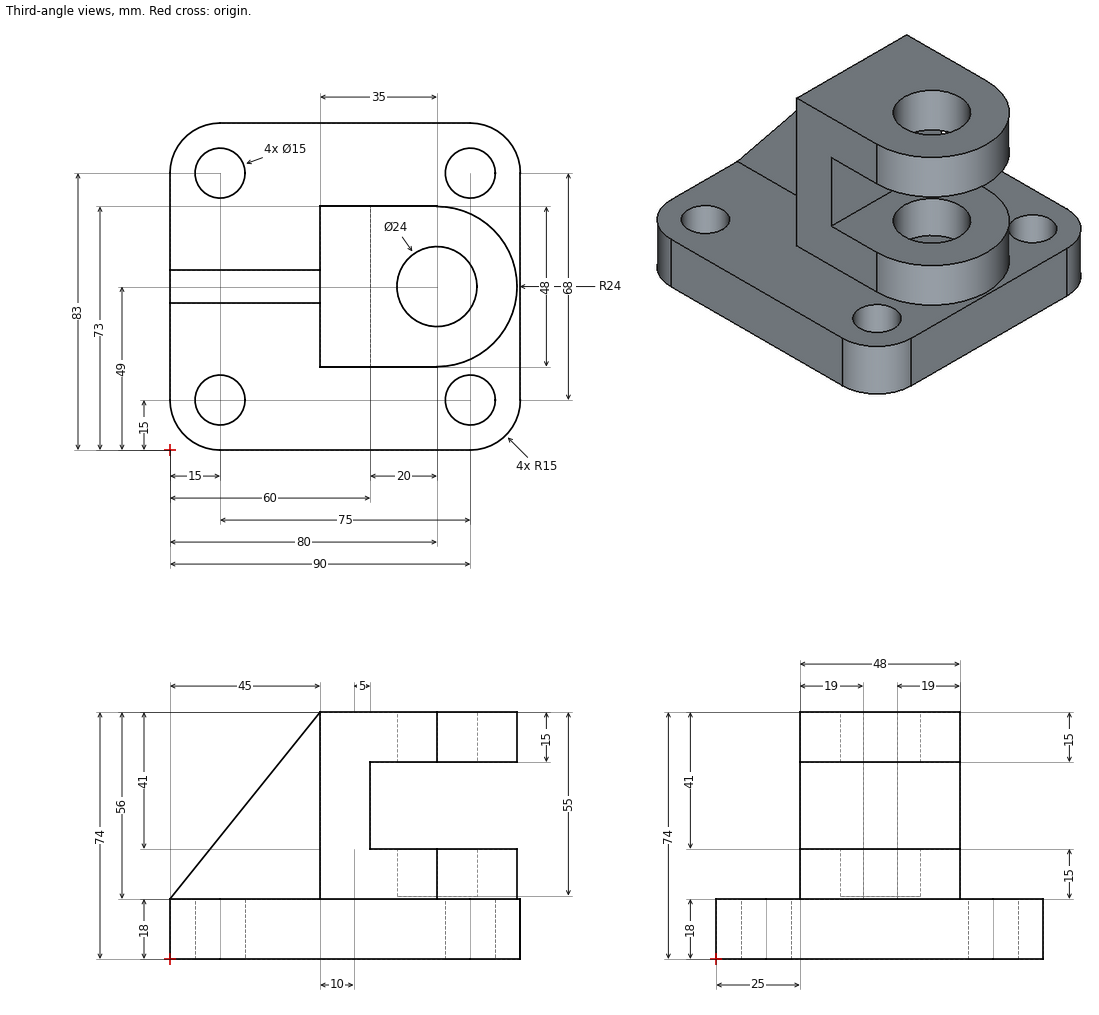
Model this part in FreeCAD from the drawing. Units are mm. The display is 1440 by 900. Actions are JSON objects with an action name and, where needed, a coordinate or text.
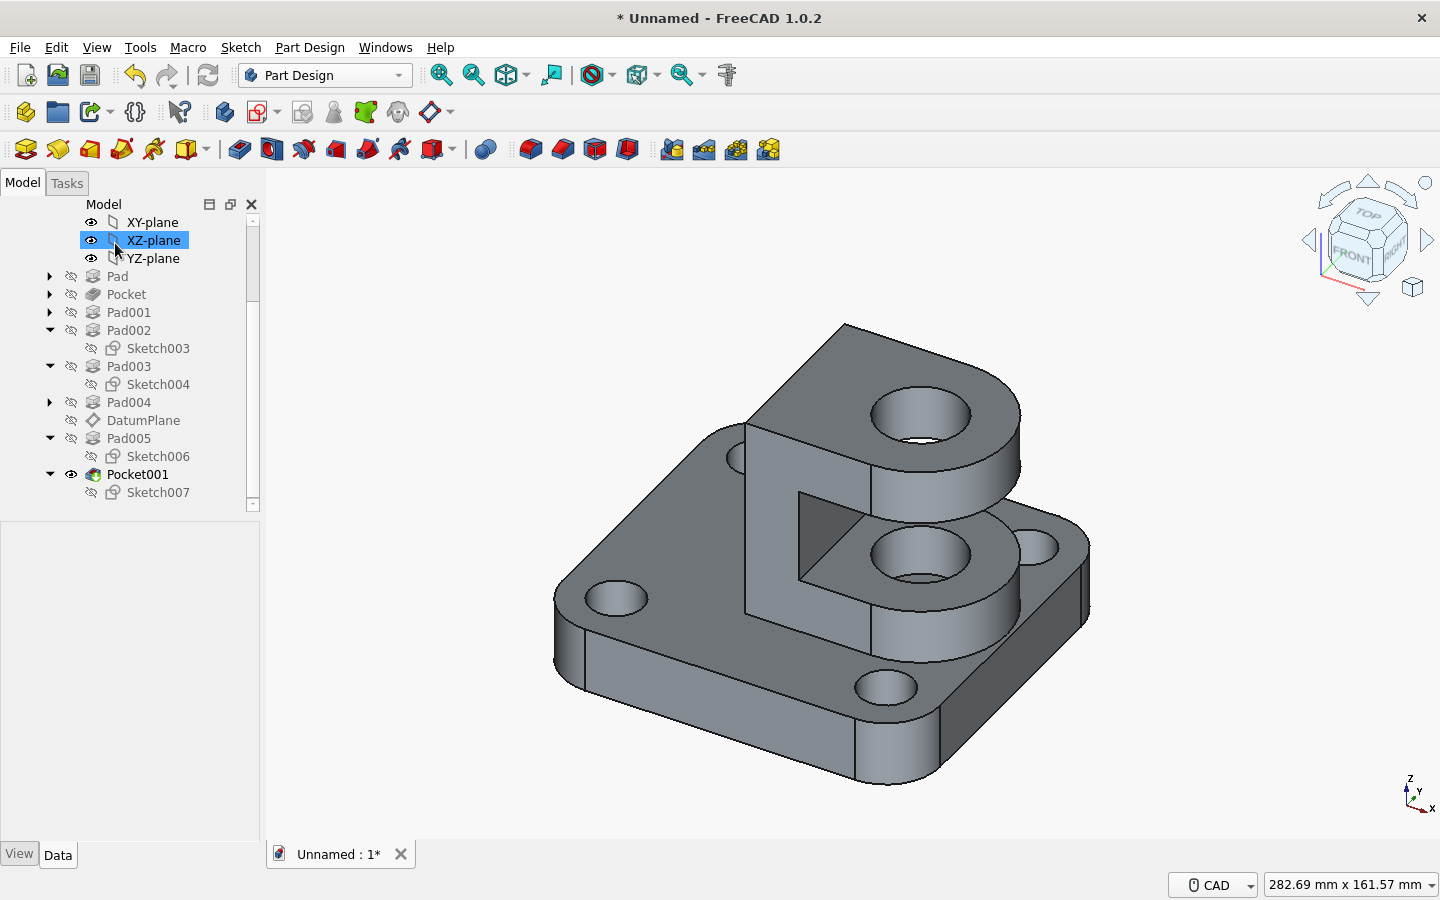
{"action": "left_click", "coordinate": [772, 472]}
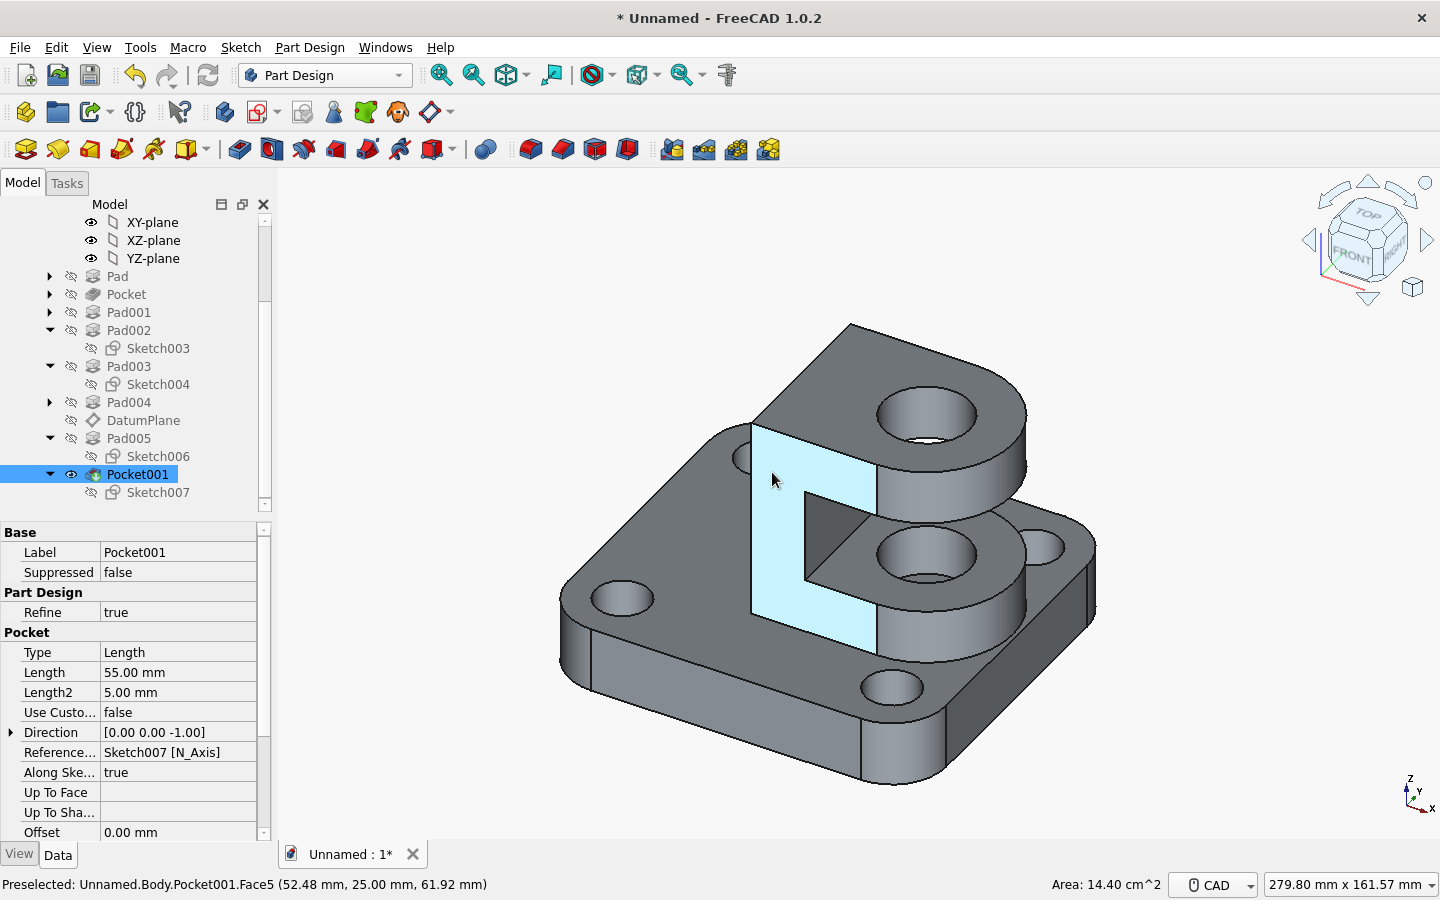
{"action": "left_click", "coordinate": [258, 112]}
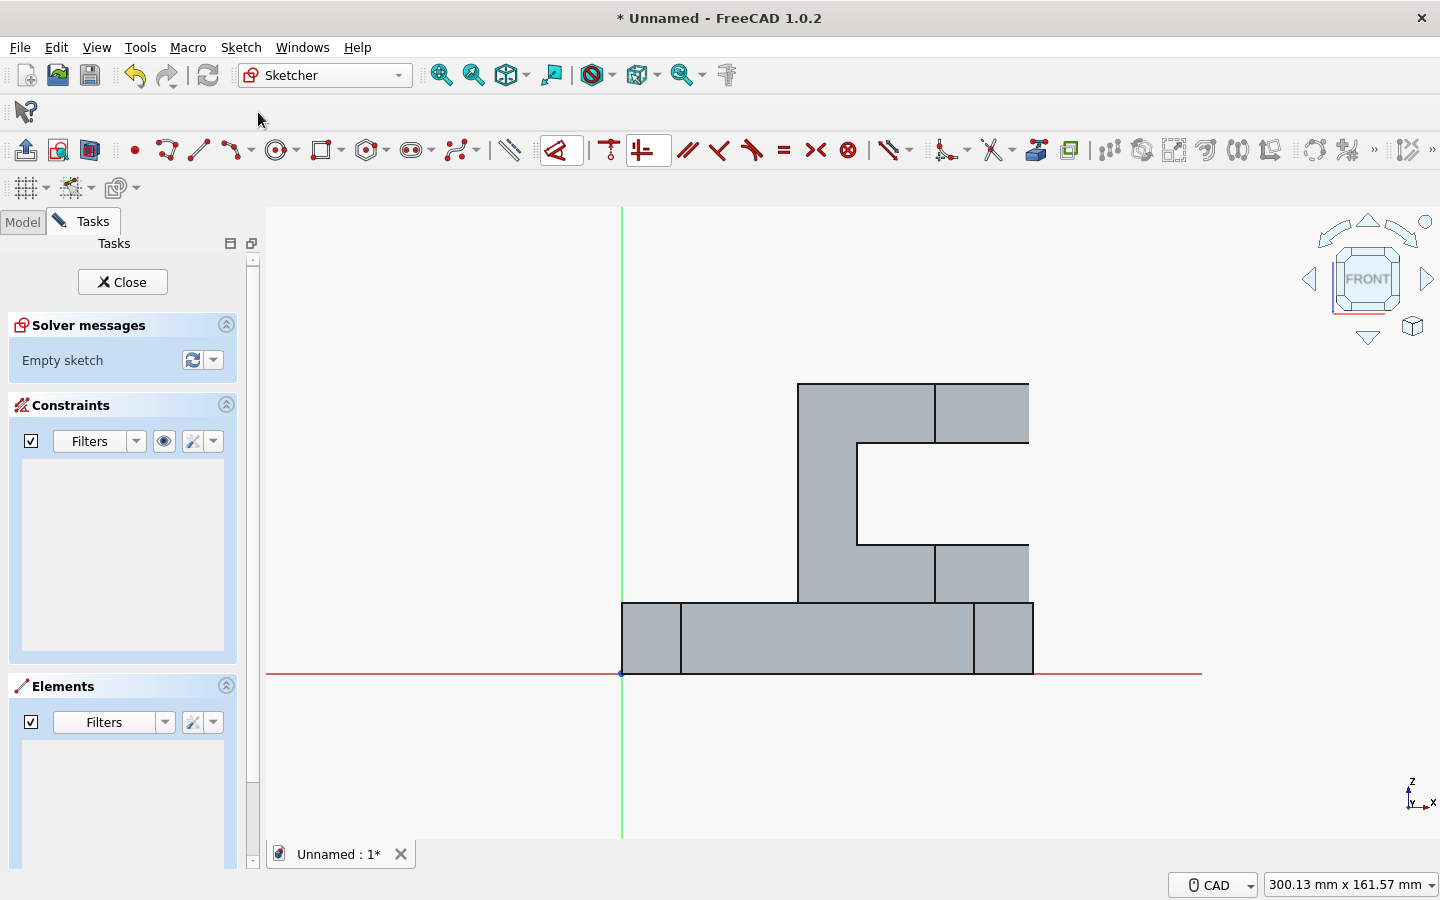
{"action": "scroll", "coordinate": [558, 541], "scroll_direction": "up", "scroll_amount": 2}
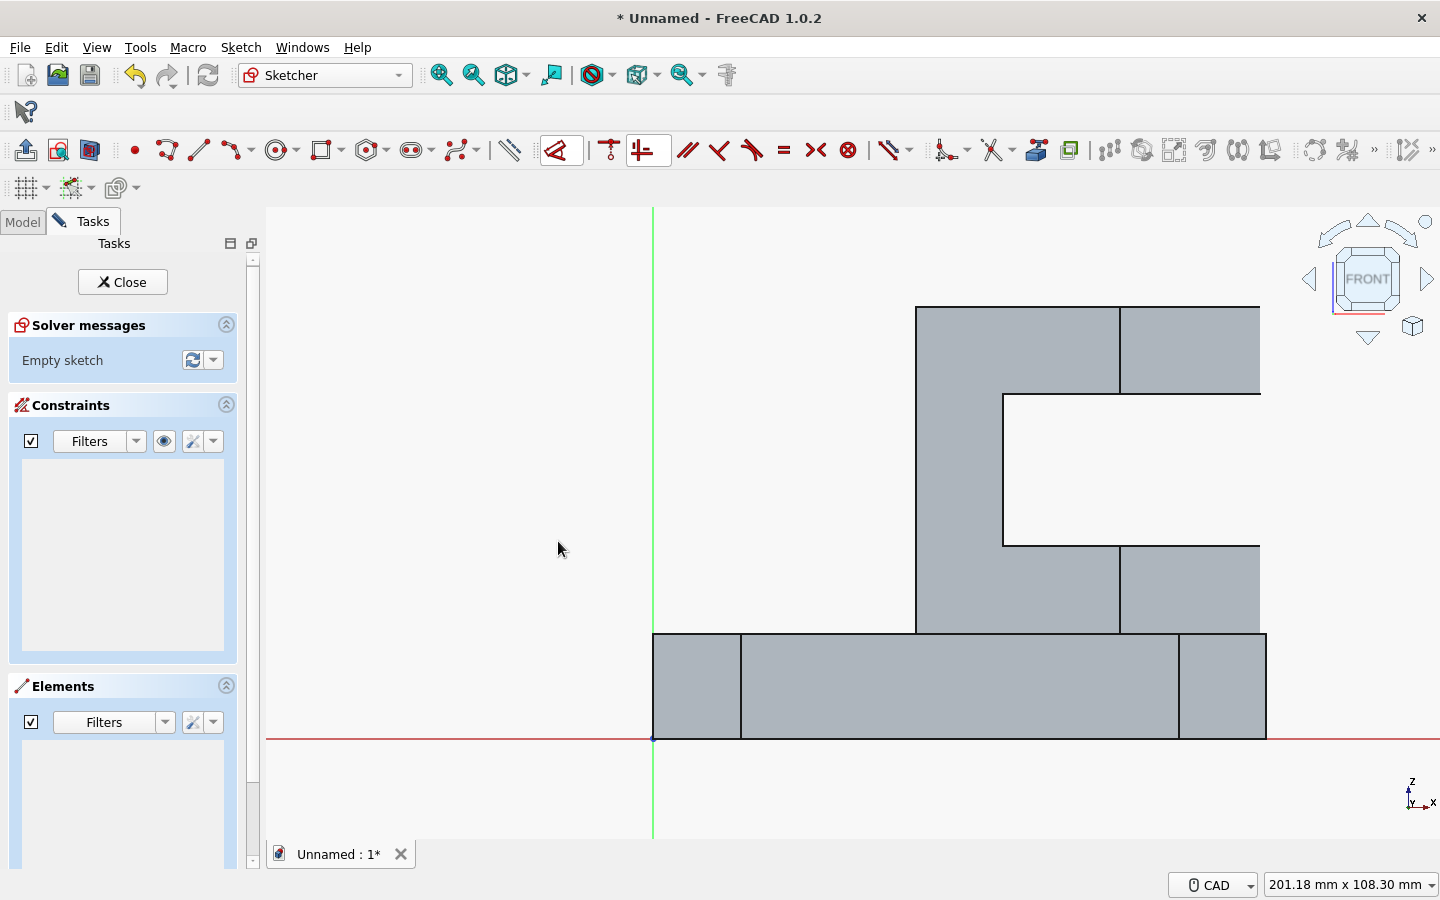
{"action": "left_click", "coordinate": [168, 150]}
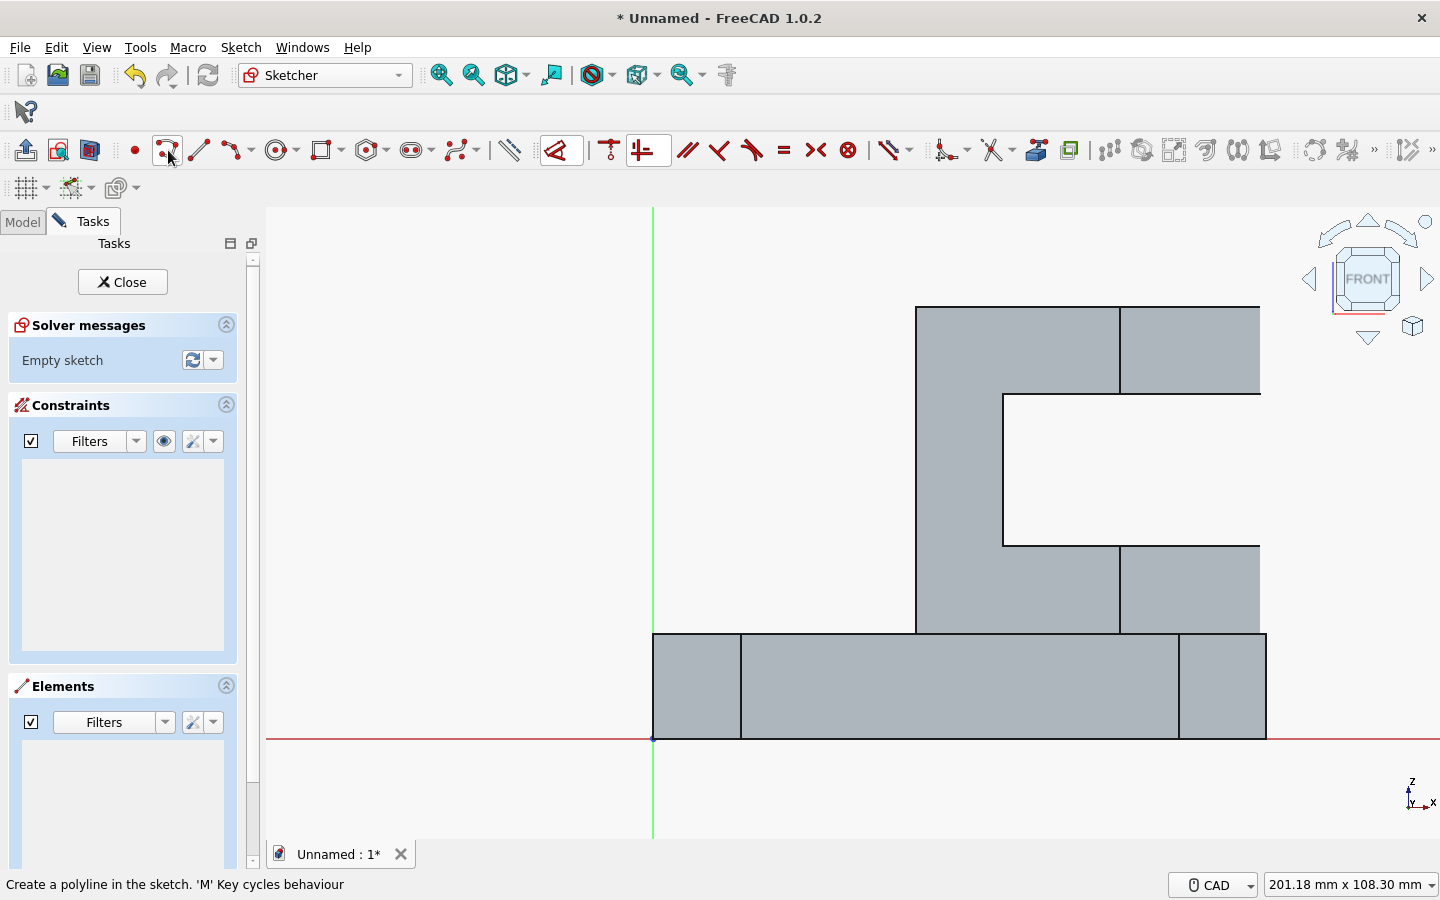
{"action": "left_click", "coordinate": [653, 634]}
{"action": "left_click", "coordinate": [916, 634]}
{"action": "left_click", "coordinate": [916, 307]}
{"action": "left_click", "coordinate": [653, 635]}
{"action": "key", "text": "Escape"}
{"action": "key", "text": "Escape"}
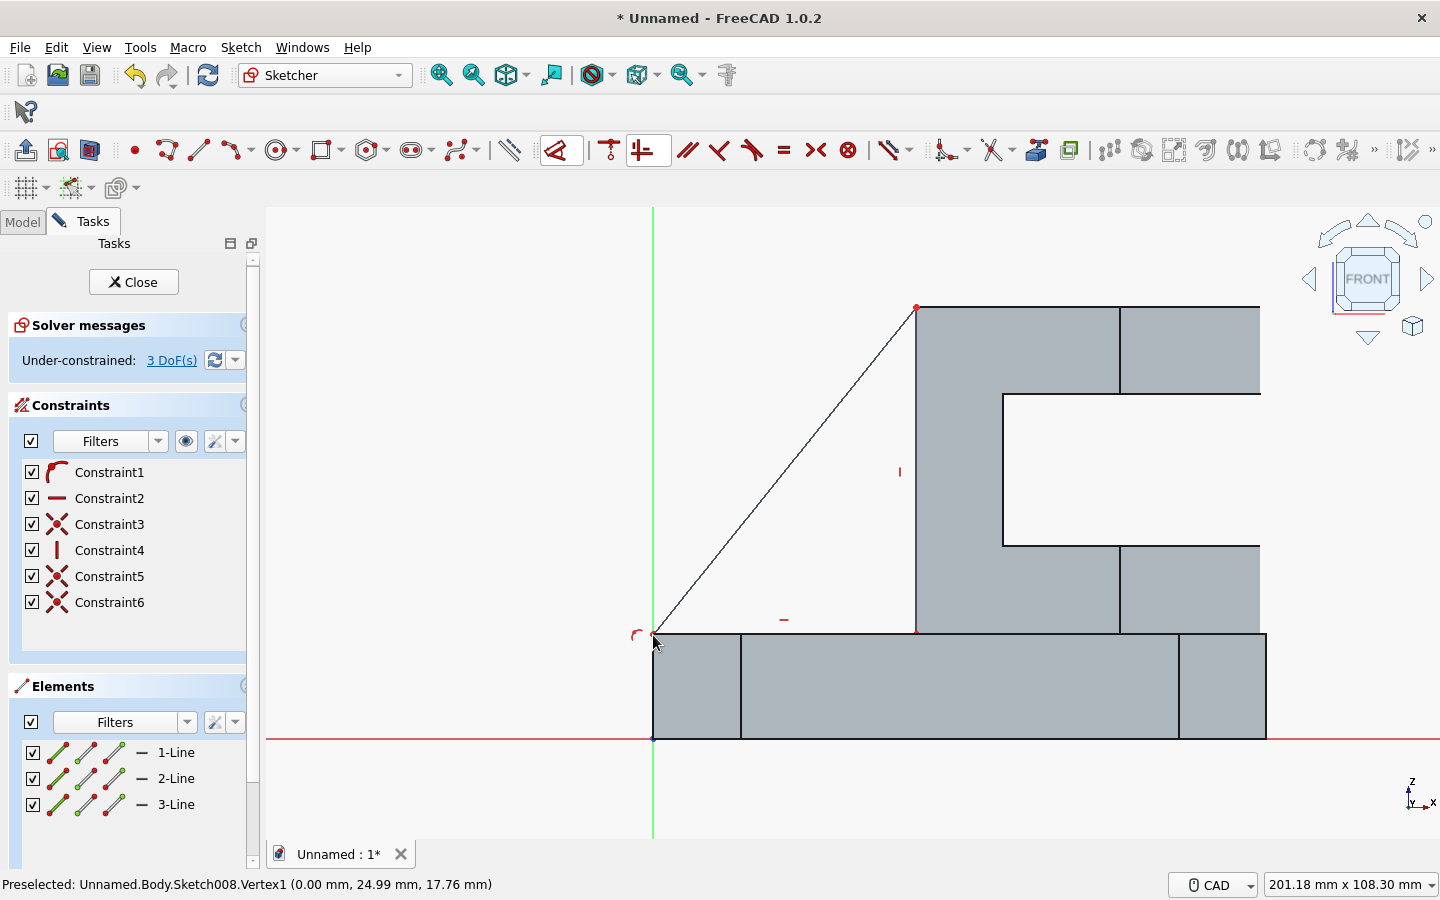
{"action": "left_click", "coordinate": [732, 635]}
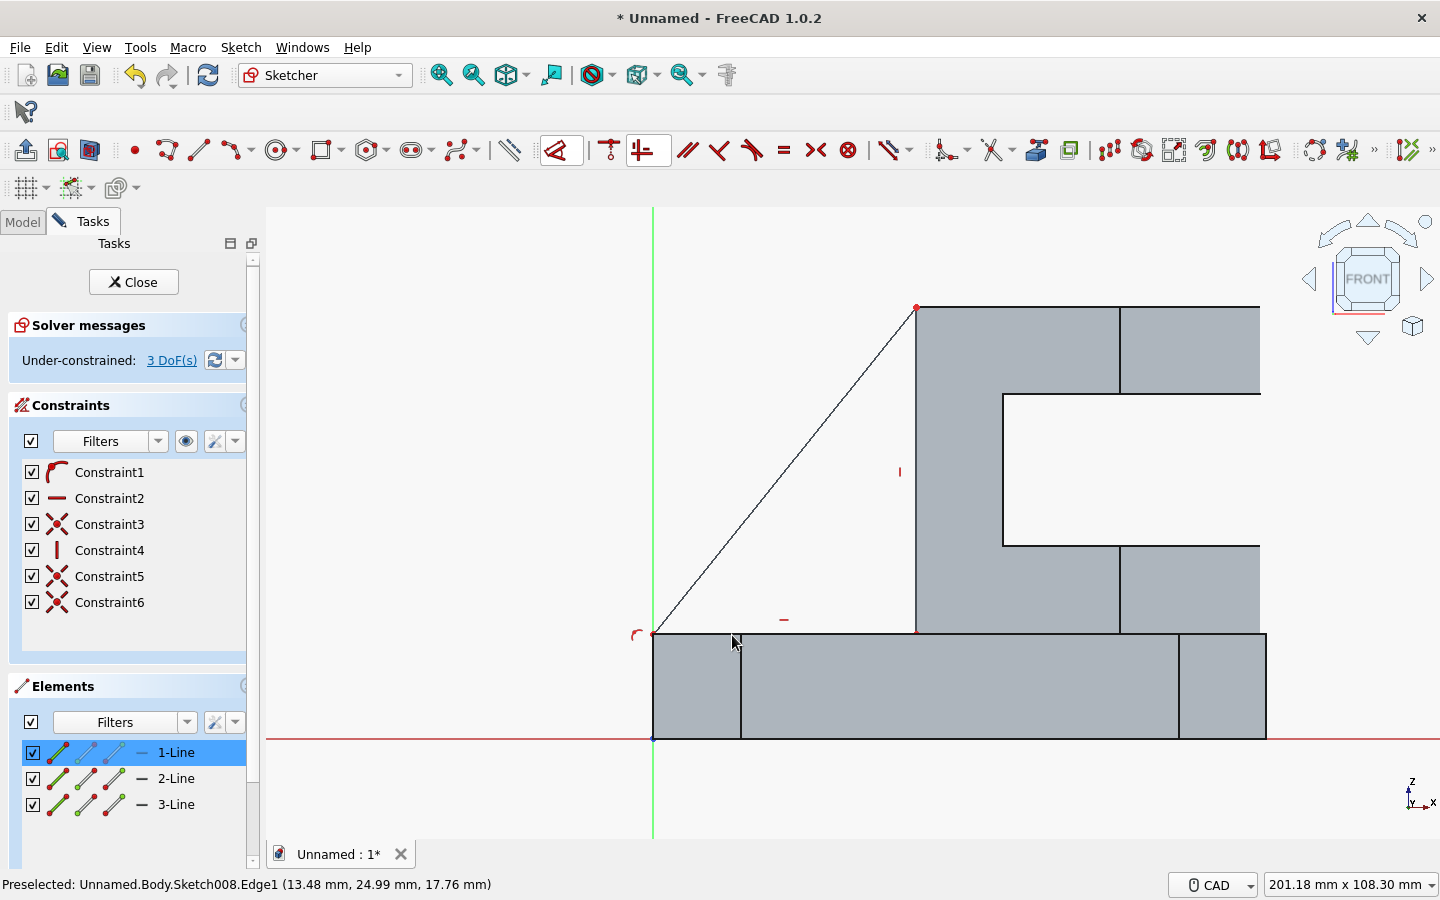
{"action": "left_click", "coordinate": [578, 150]}